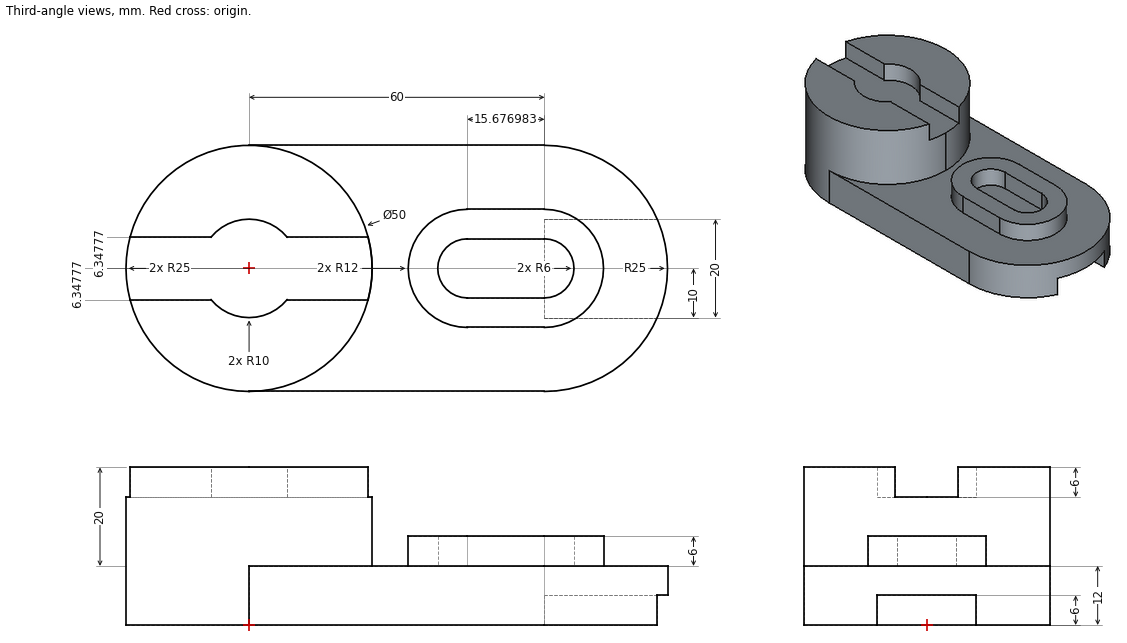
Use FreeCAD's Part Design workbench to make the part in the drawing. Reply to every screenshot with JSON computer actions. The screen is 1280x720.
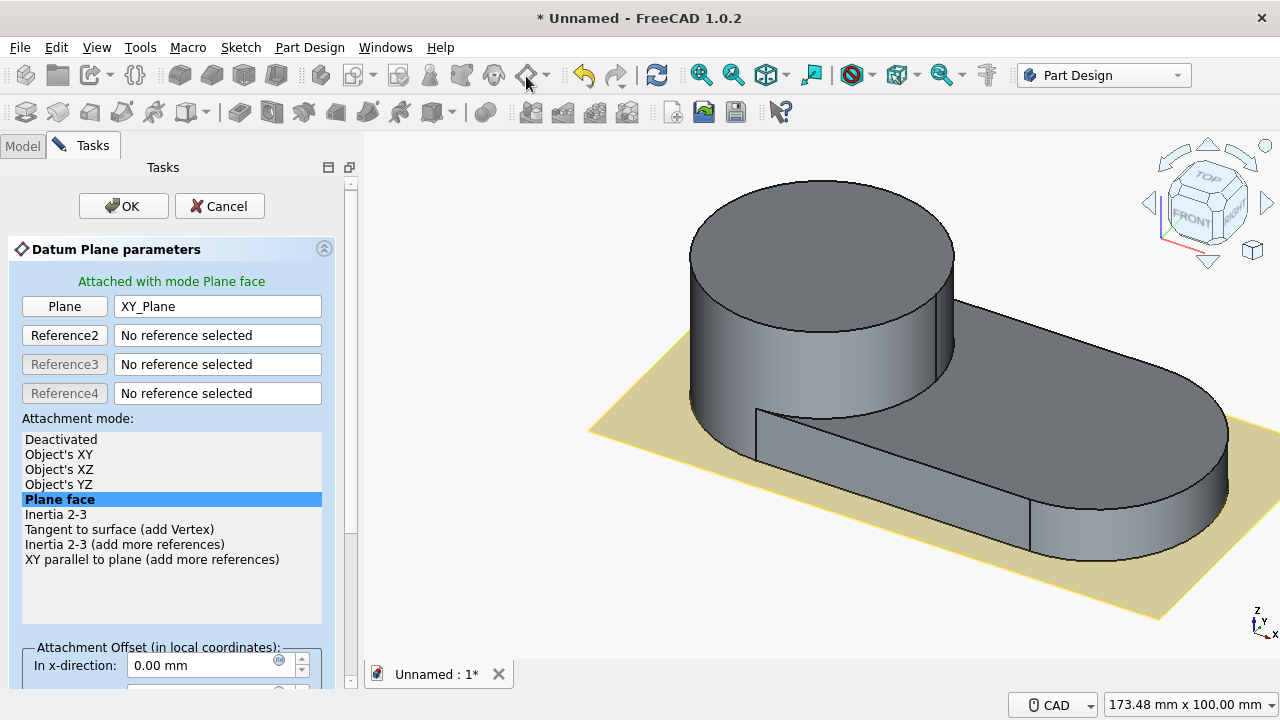
{"action": "scroll", "coordinate": [351, 432], "scroll_direction": "down", "scroll_amount": 2}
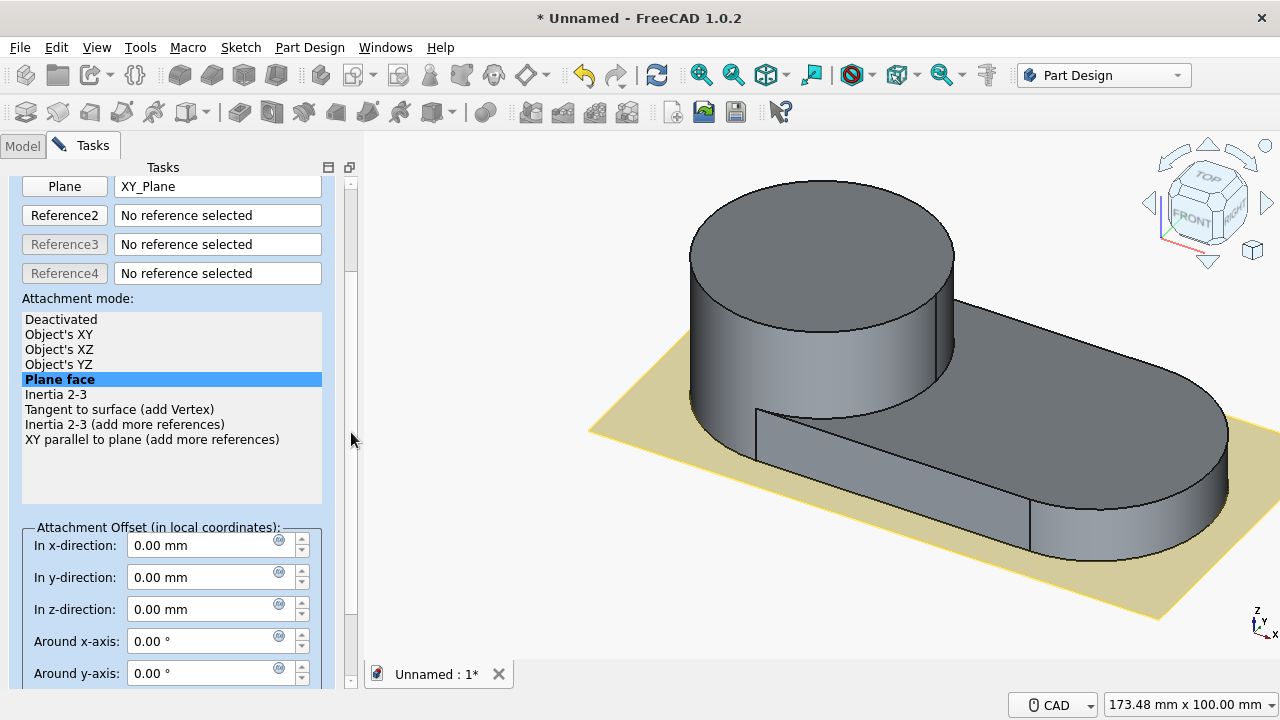
{"action": "triple_click", "coordinate": [210, 609]}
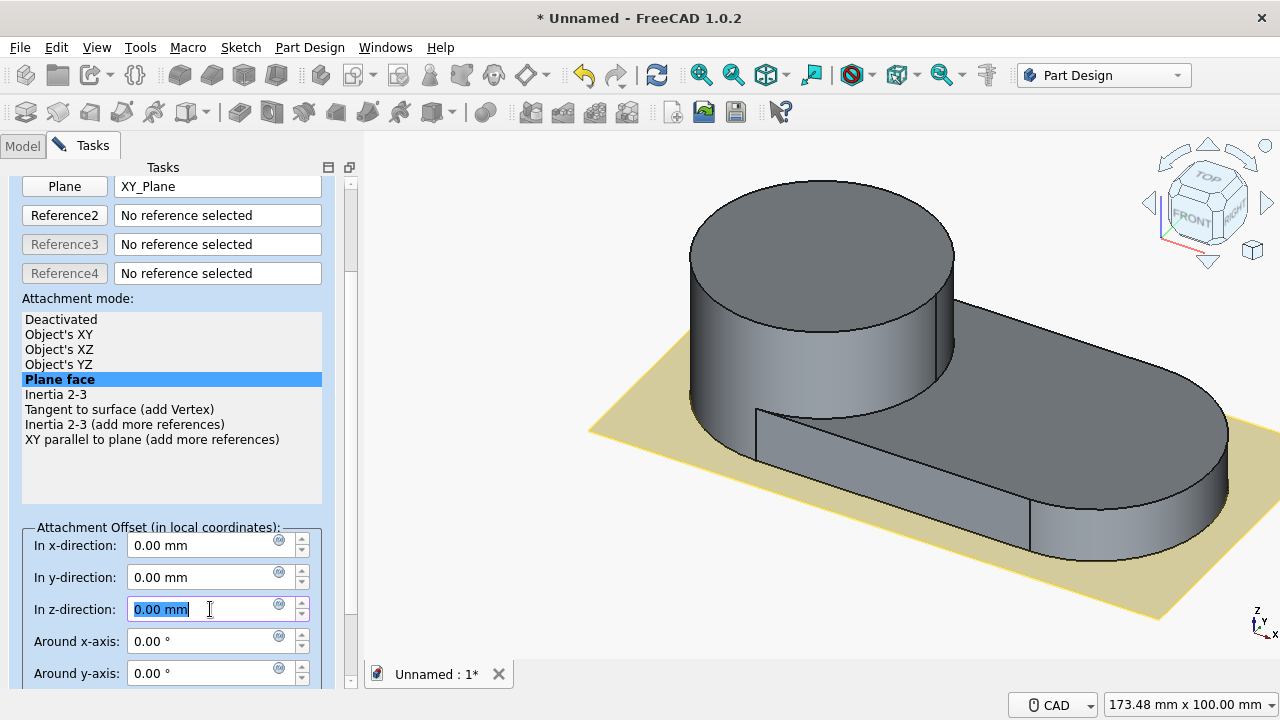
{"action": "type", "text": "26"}
{"action": "key", "text": "Tab"}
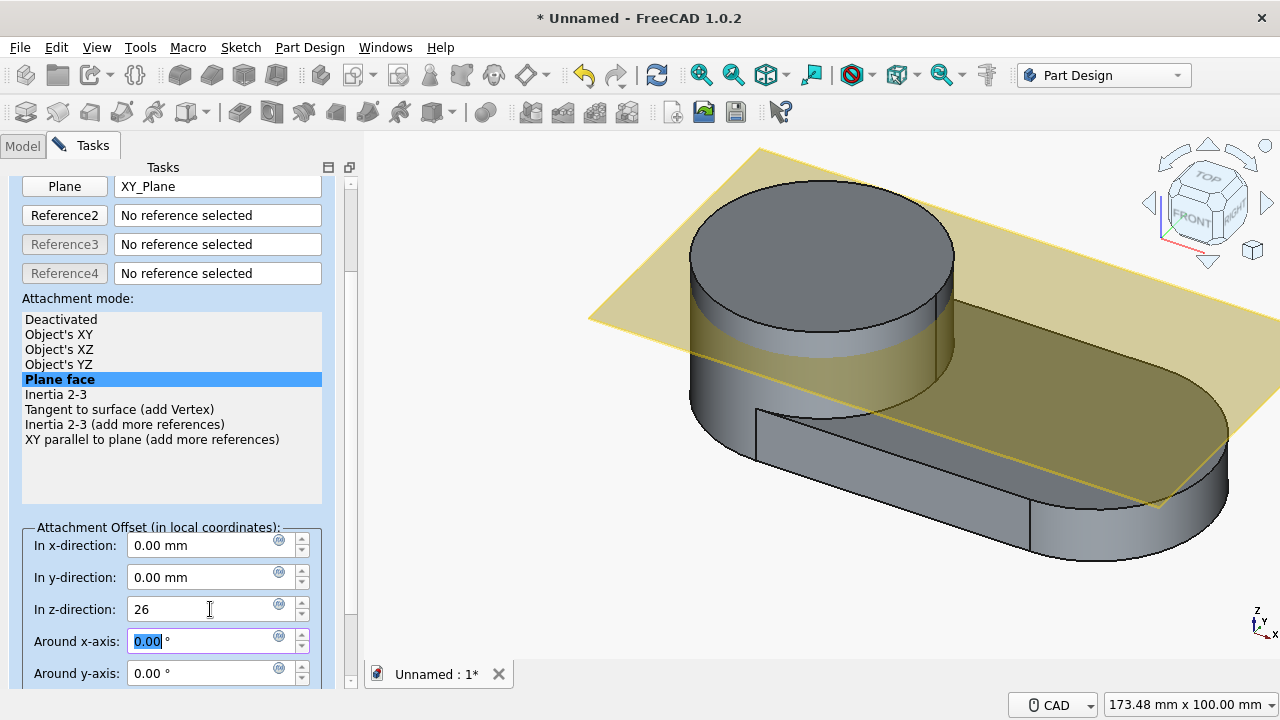
{"action": "scroll", "coordinate": [351, 432], "scroll_direction": "up", "scroll_amount": 3}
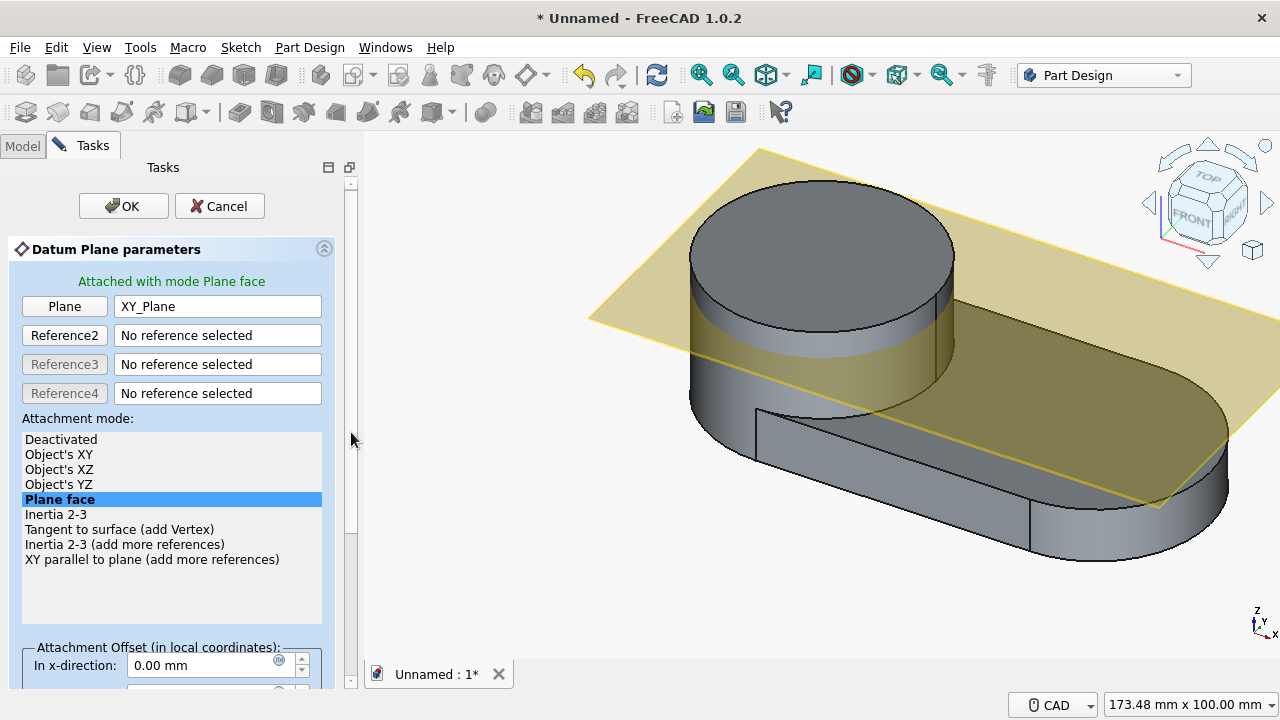
{"action": "left_click", "coordinate": [124, 206]}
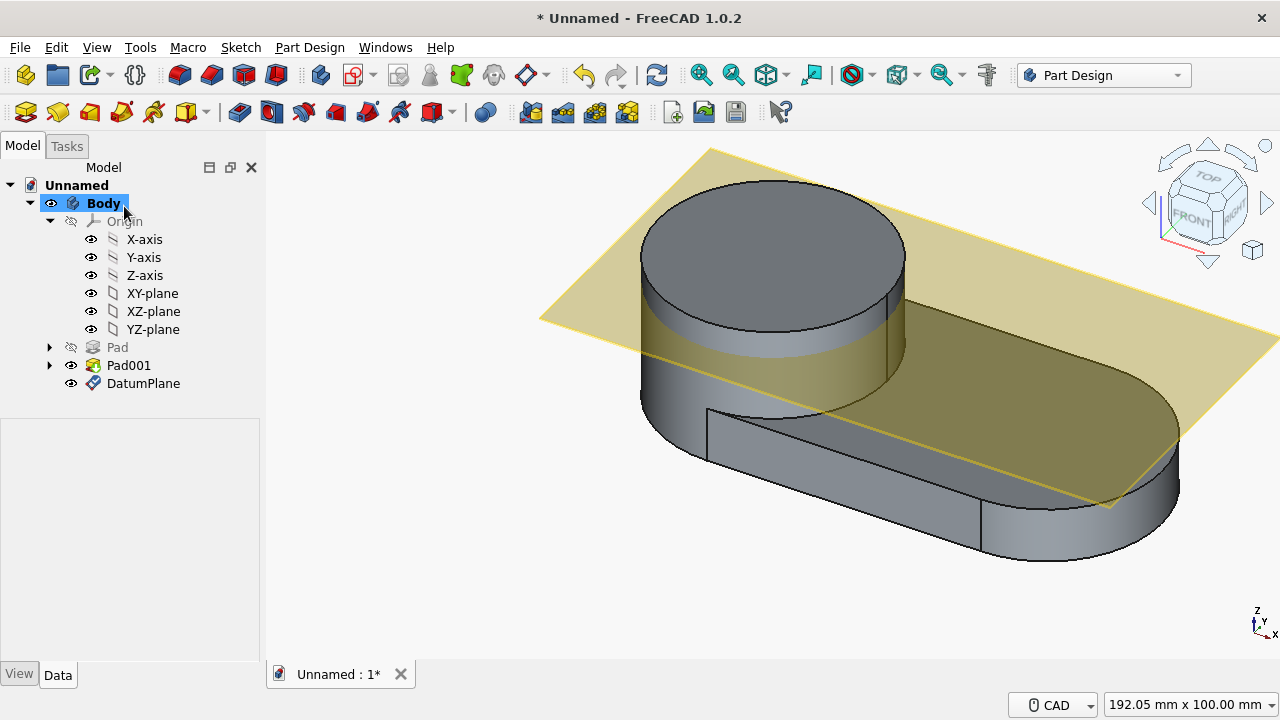
{"action": "left_click", "coordinate": [116, 383]}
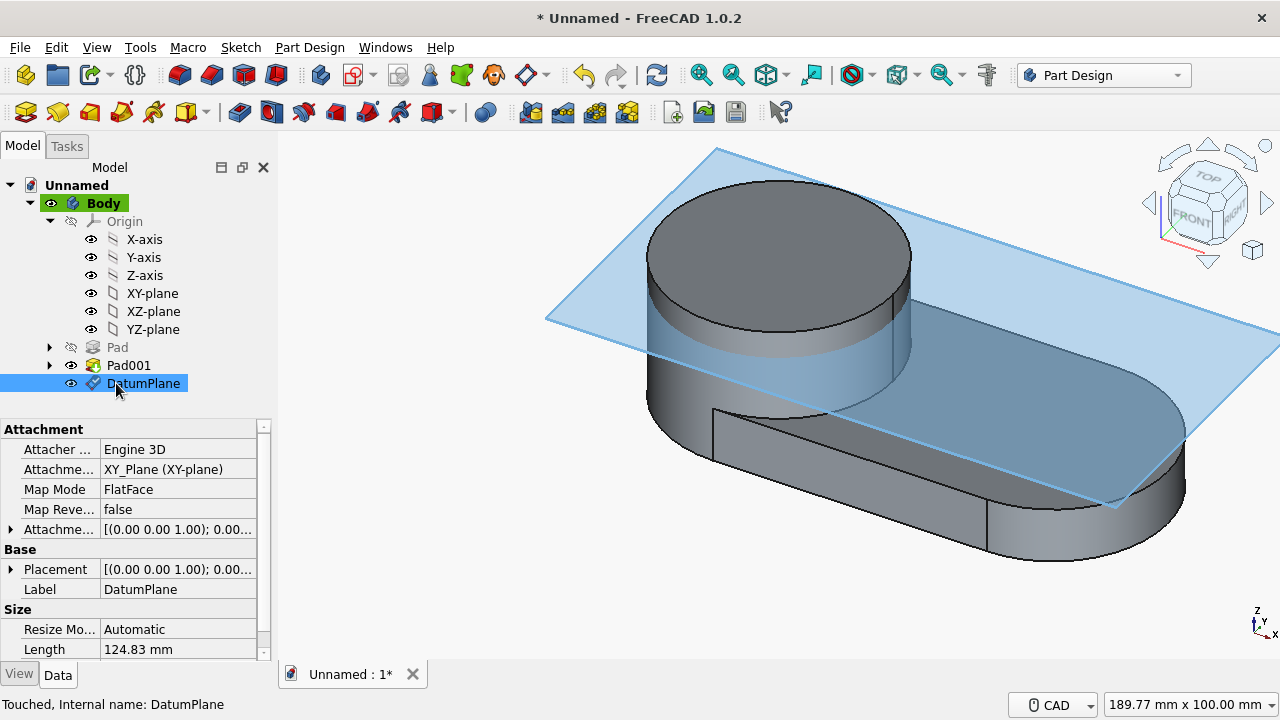
{"action": "left_click", "coordinate": [354, 76]}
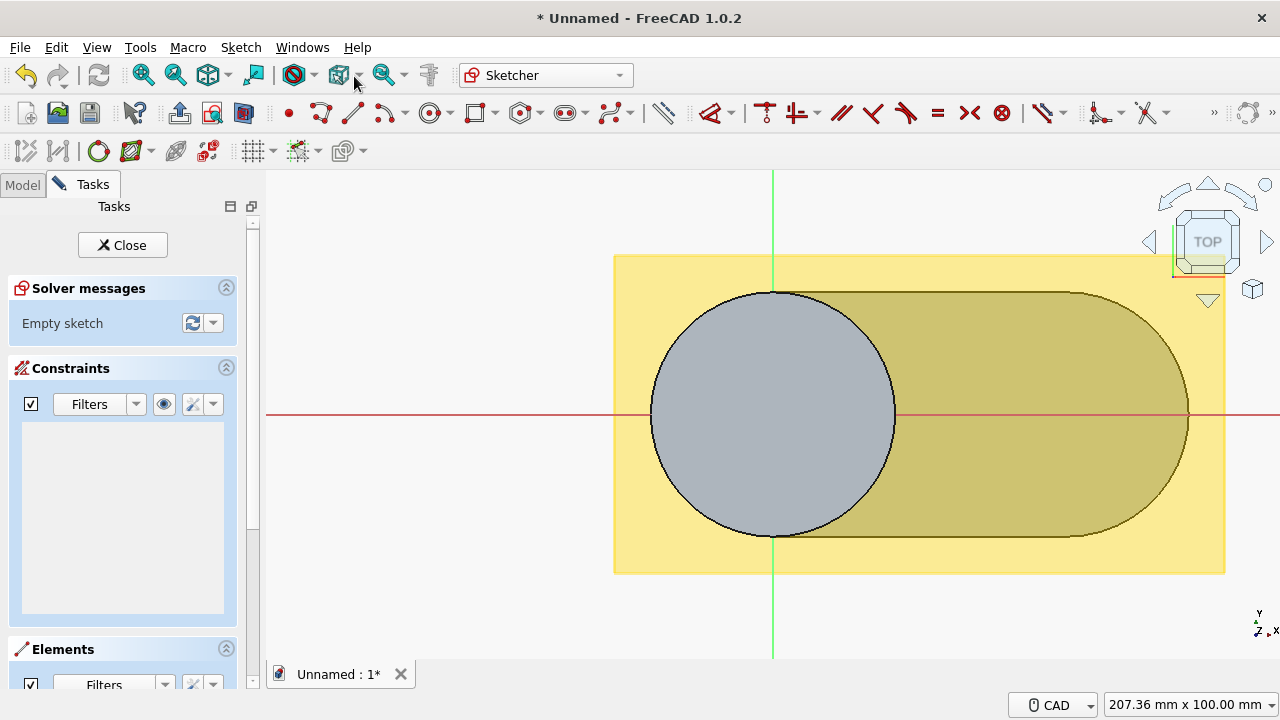
{"action": "key", "text": "q s"}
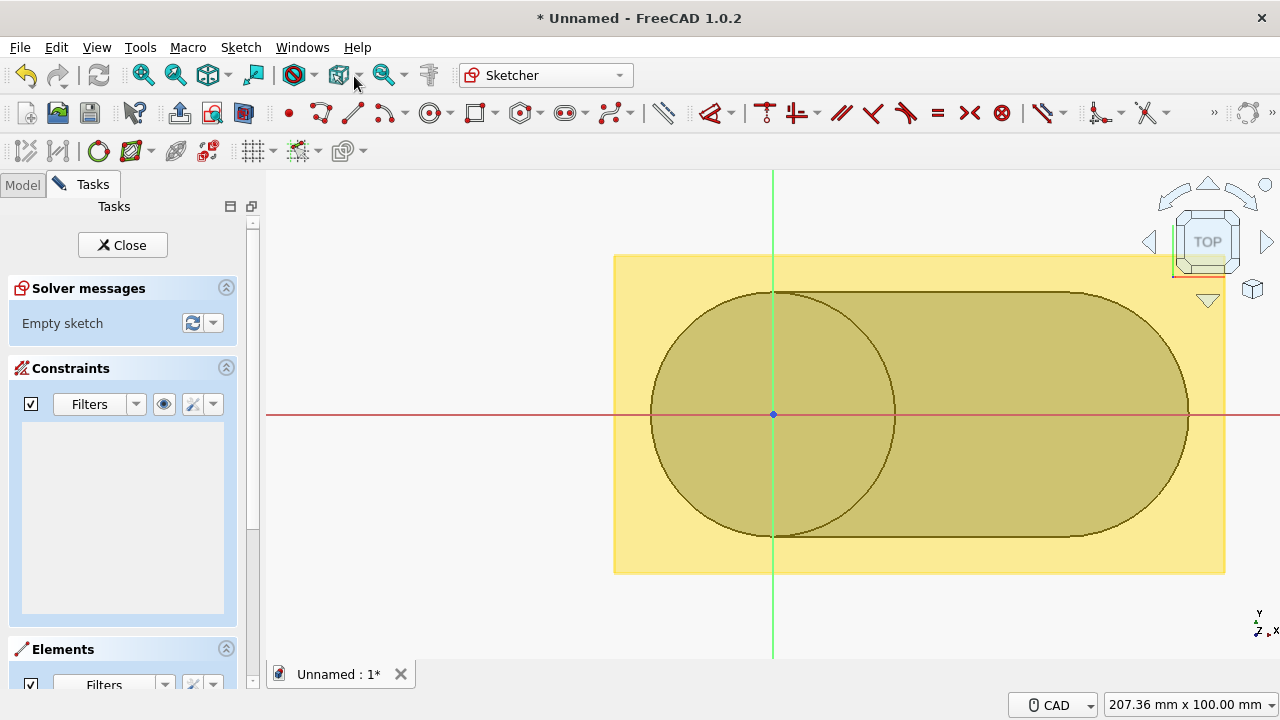
{"action": "scroll", "coordinate": [829, 414], "scroll_direction": "up", "scroll_amount": 4}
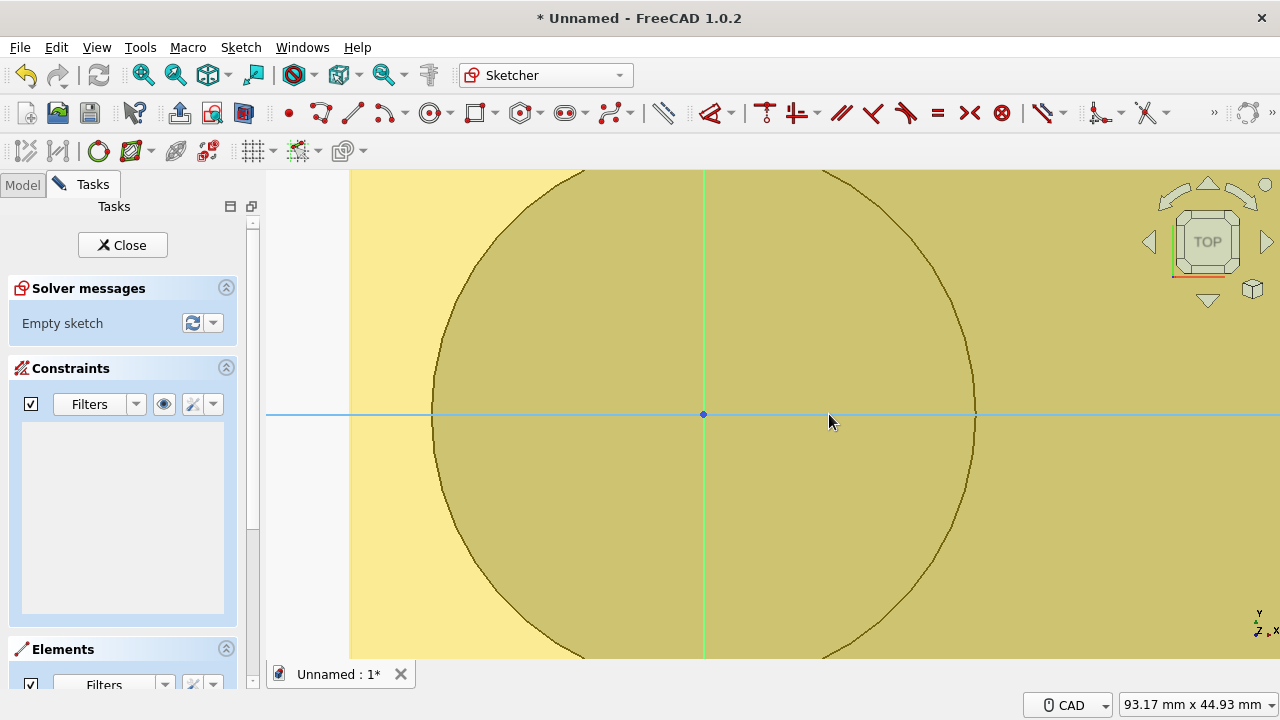
{"action": "key", "text": "g l"}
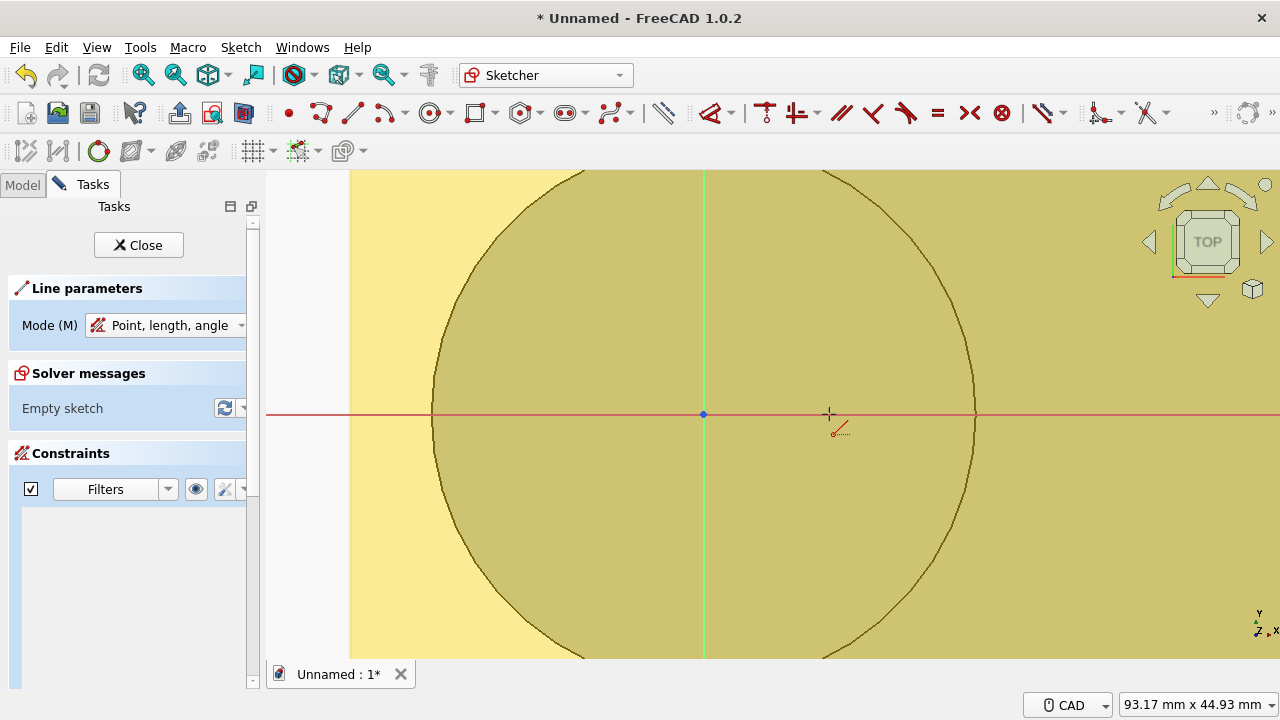
{"action": "left_click", "coordinate": [620, 345]}
{"action": "left_click", "coordinate": [441, 345]}